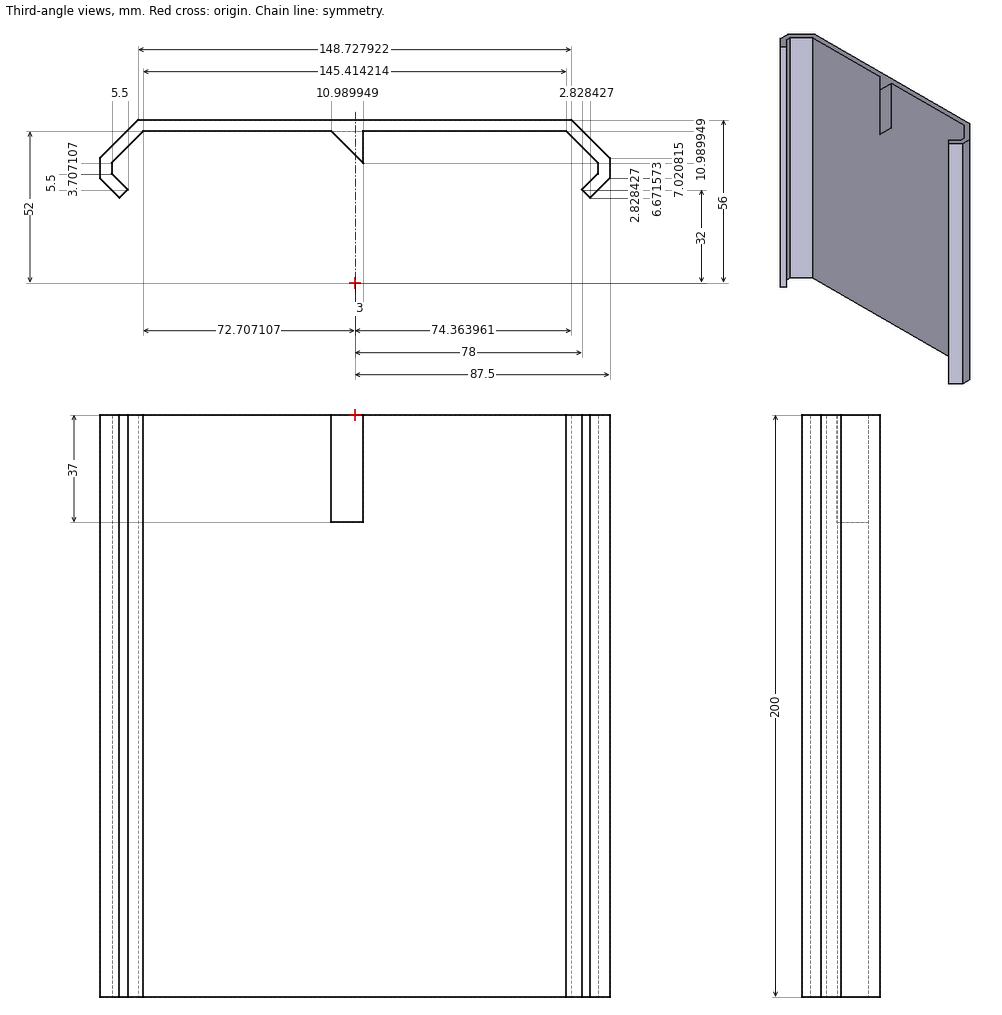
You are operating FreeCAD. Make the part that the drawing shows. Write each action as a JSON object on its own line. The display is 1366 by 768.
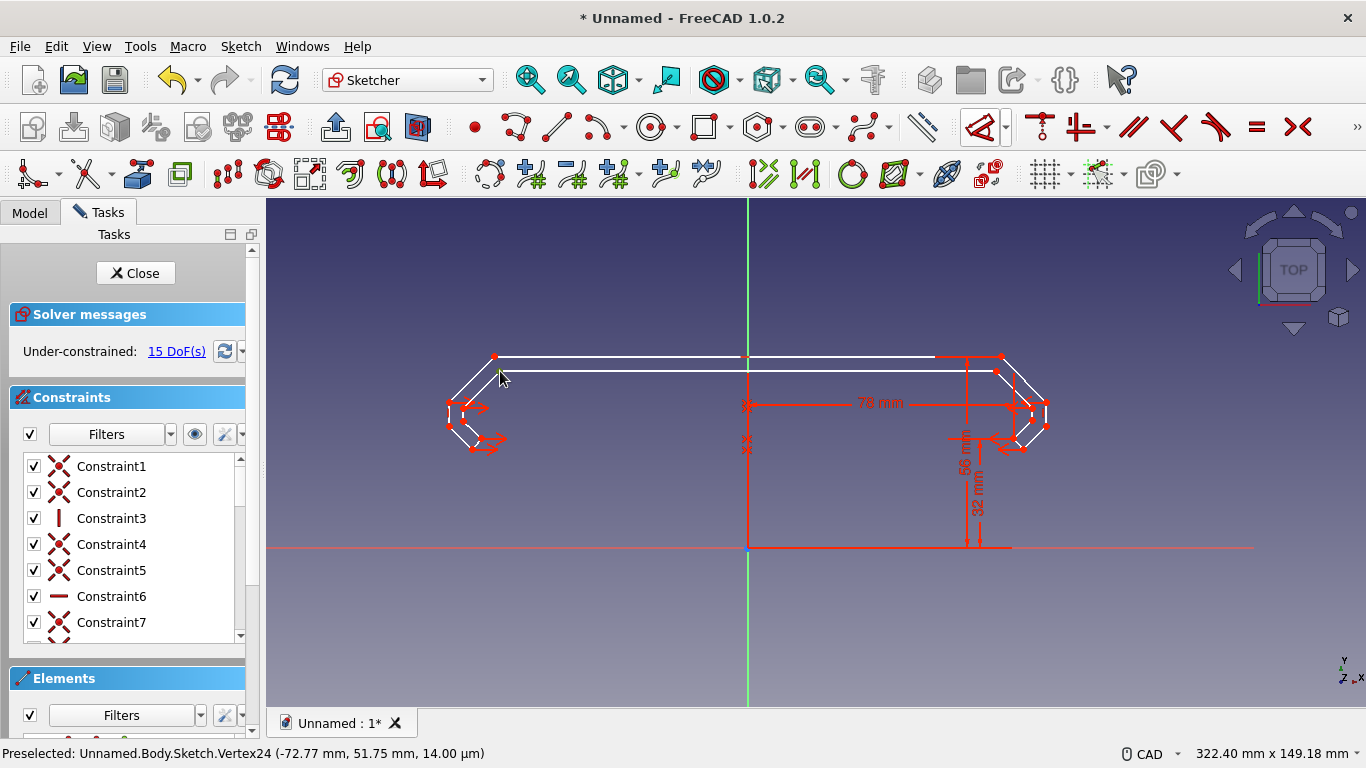
{"action": "left_click", "coordinate": [1006, 128]}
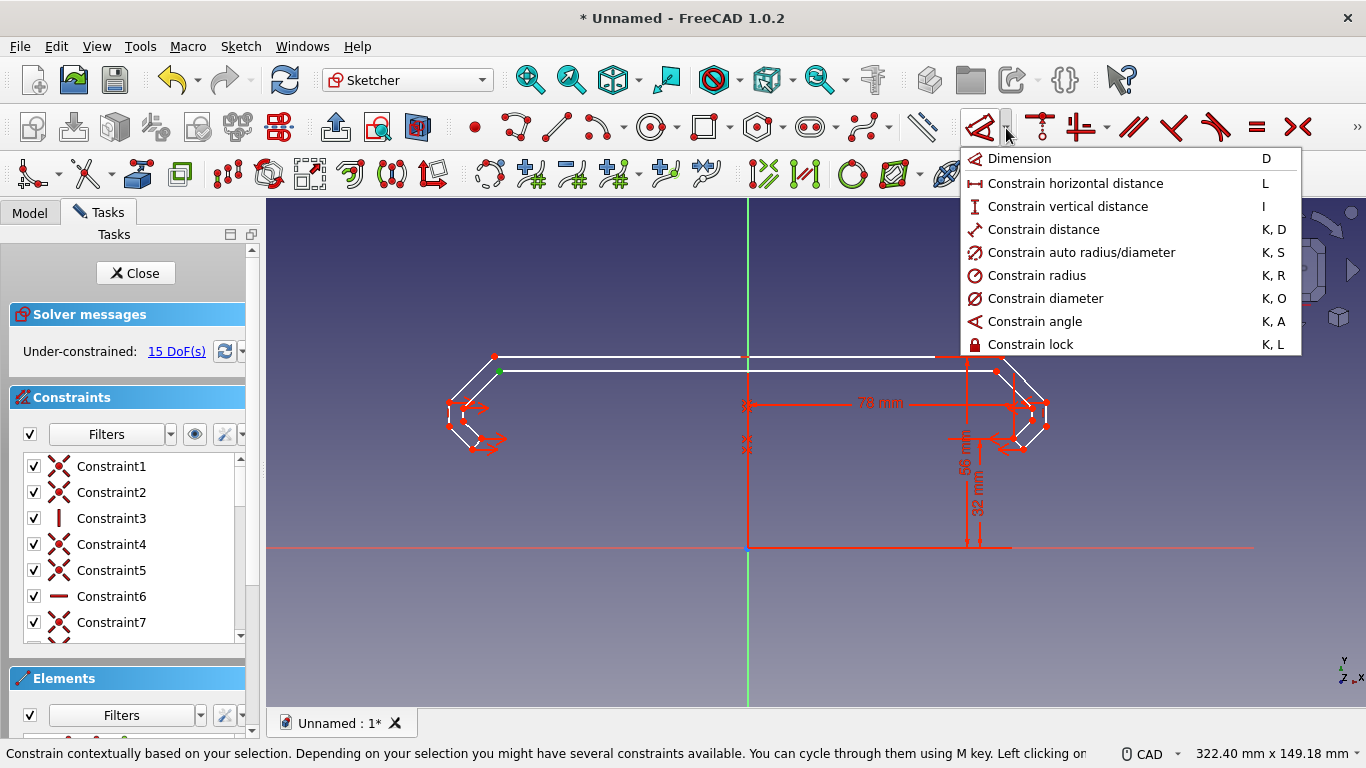
{"action": "left_click", "coordinate": [1131, 206]}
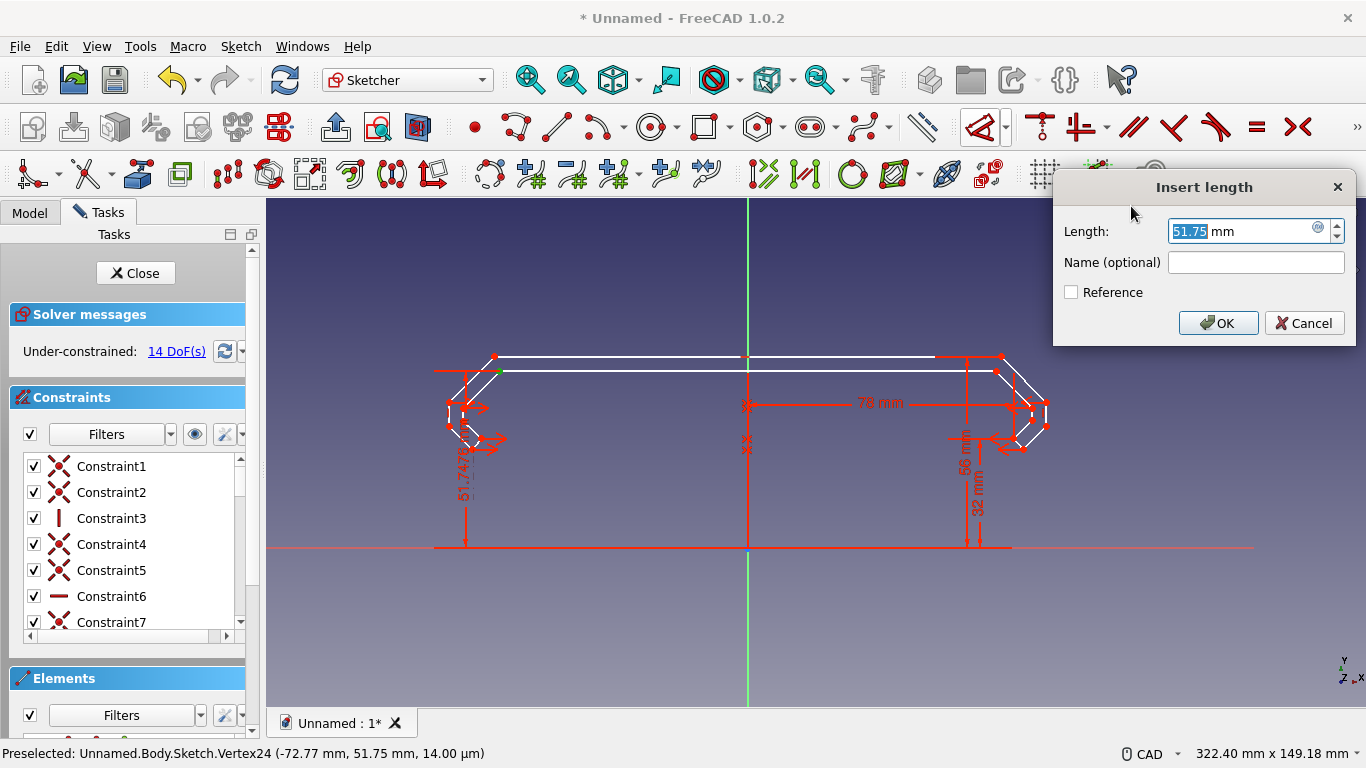
{"action": "type", "text": "52"}
{"action": "key", "text": "Return"}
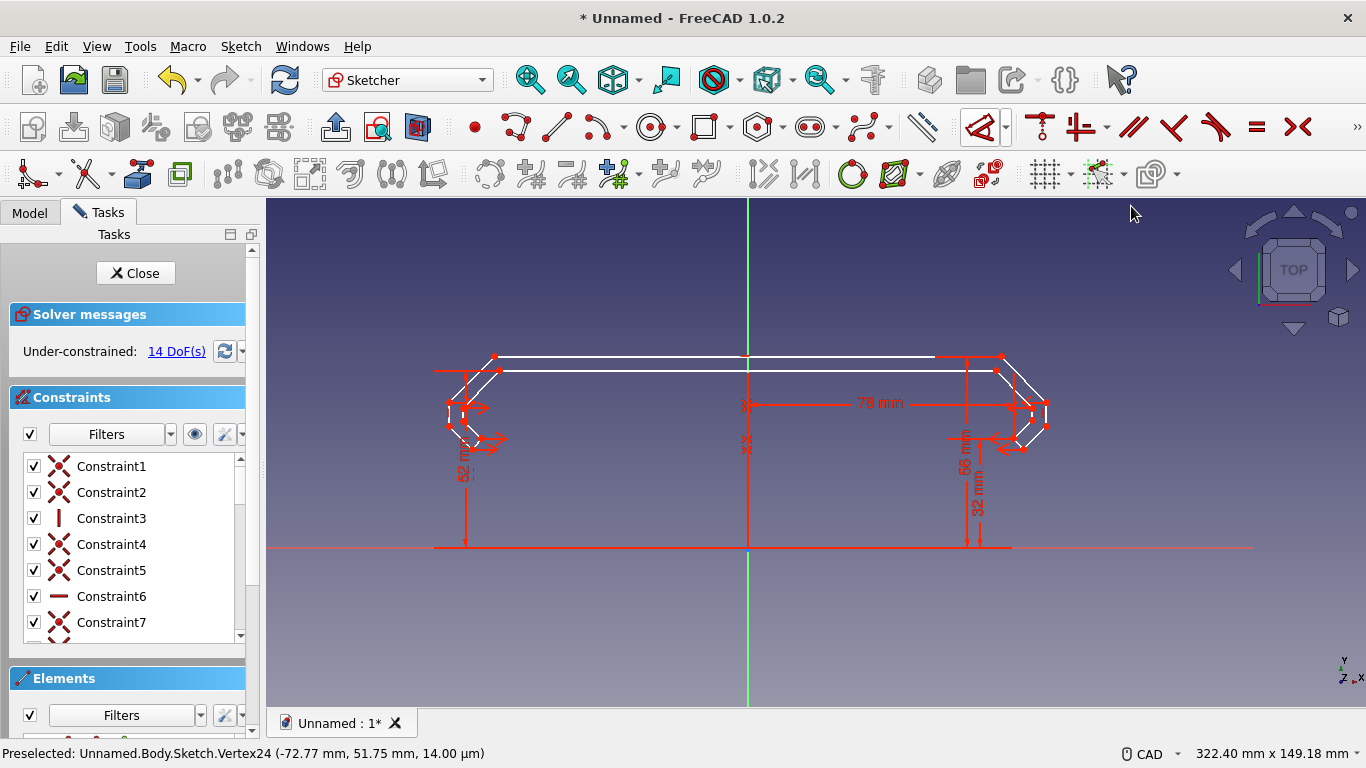
{"action": "scroll", "coordinate": [474, 432], "scroll_direction": "up", "scroll_amount": 4}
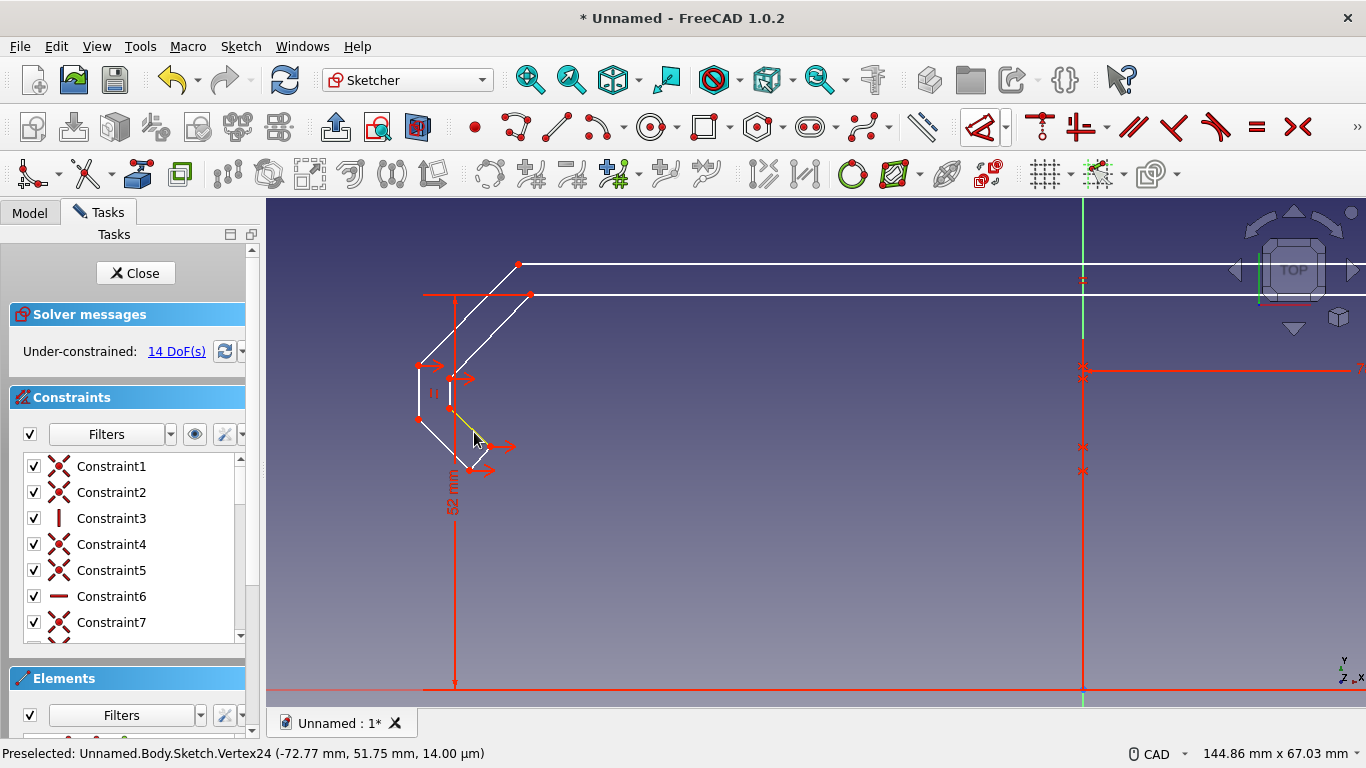
{"action": "left_click", "coordinate": [474, 431]}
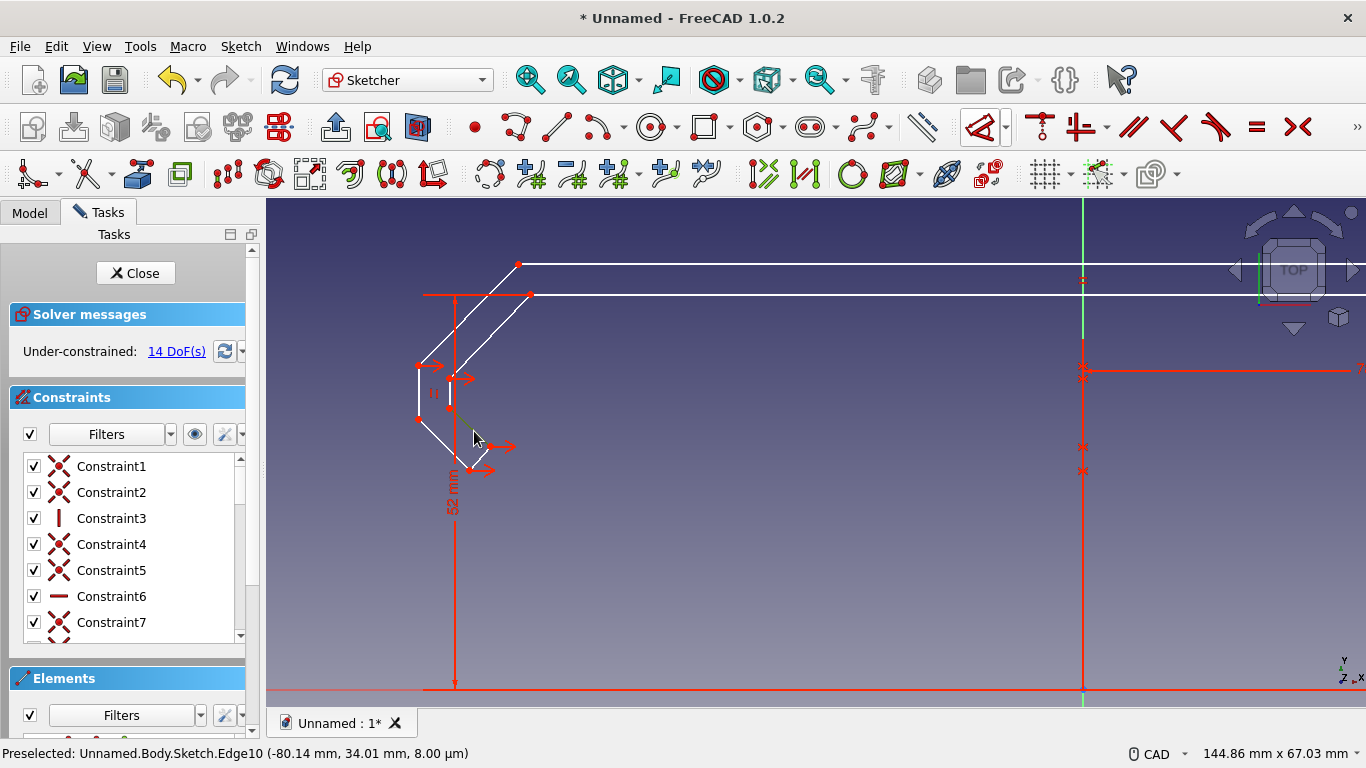
{"action": "left_click", "coordinate": [1006, 128]}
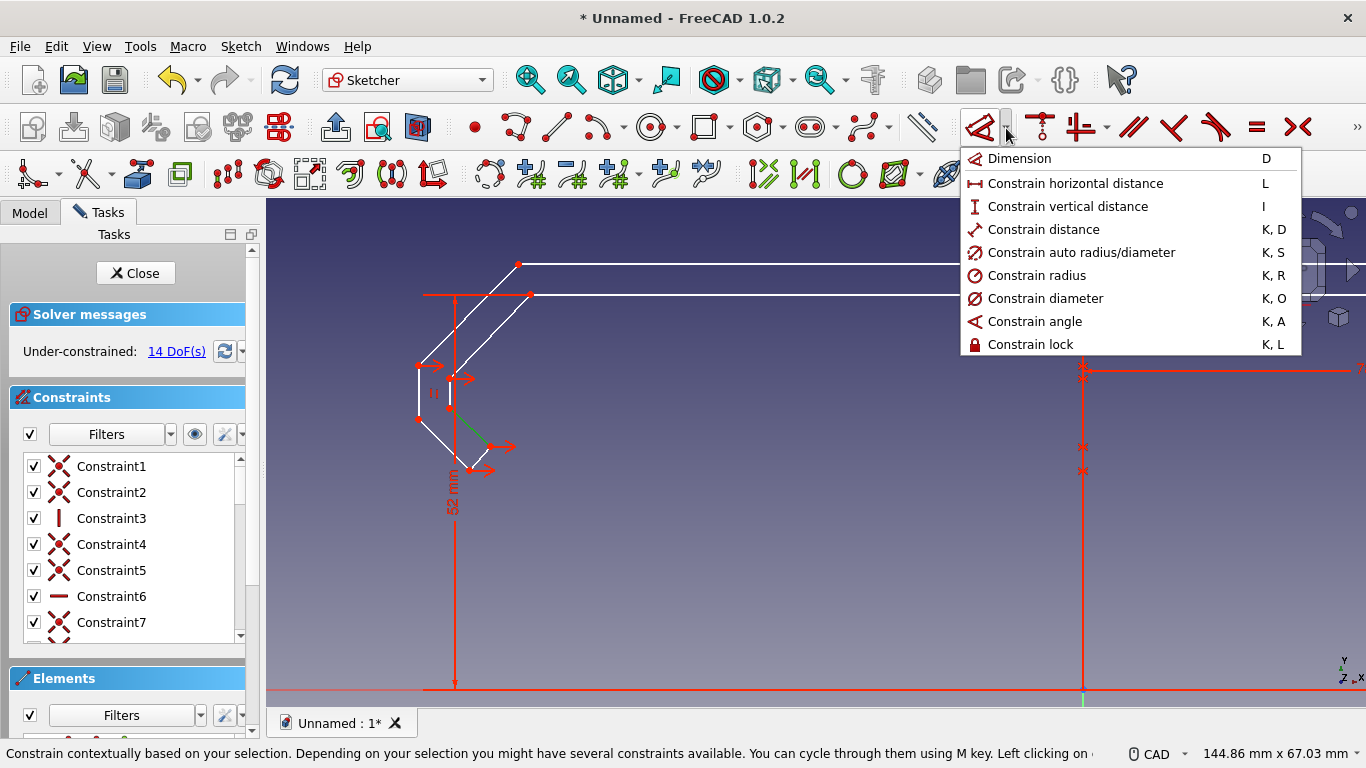
{"action": "left_click", "coordinate": [1131, 184]}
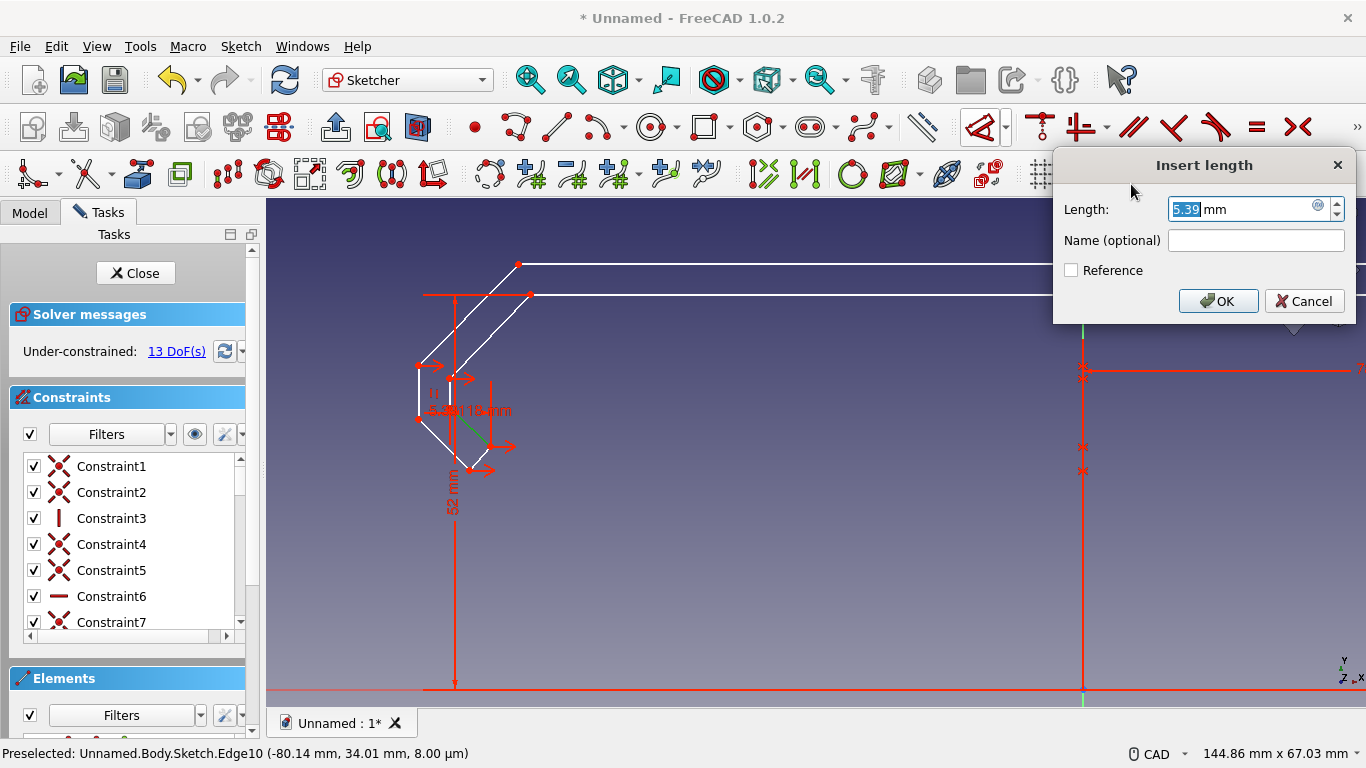
{"action": "type", "text": "5.5"}
{"action": "key", "text": "Return"}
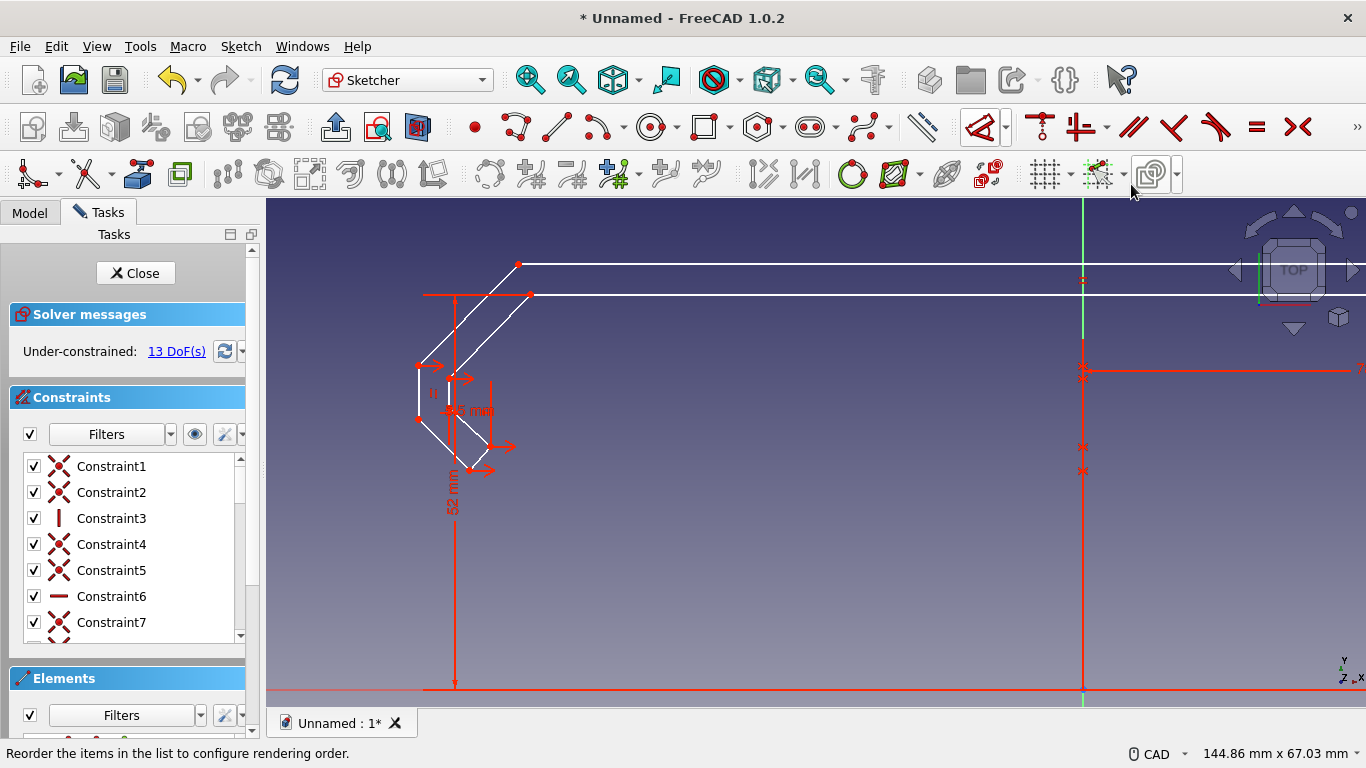
{"action": "left_click", "coordinate": [478, 435]}